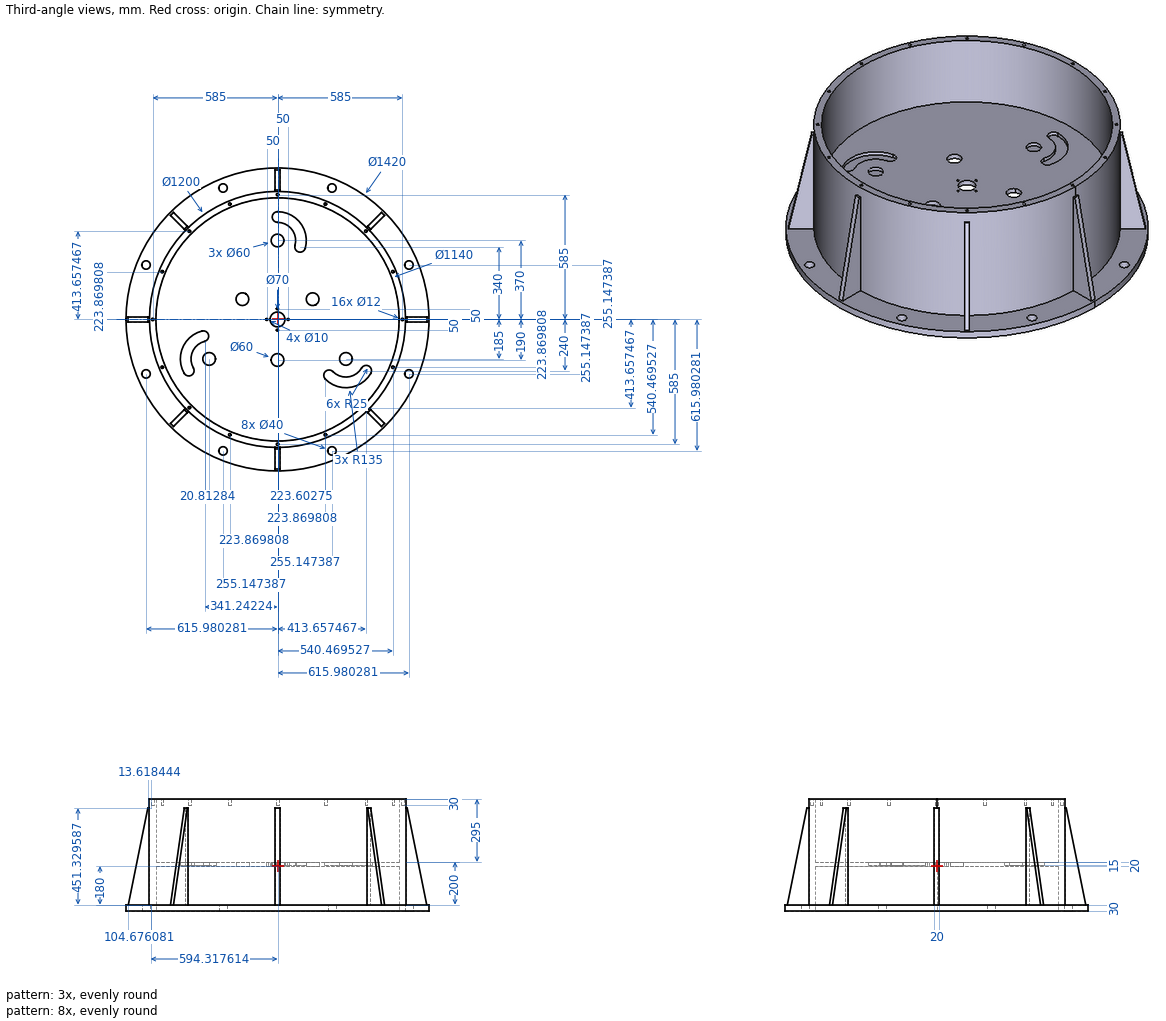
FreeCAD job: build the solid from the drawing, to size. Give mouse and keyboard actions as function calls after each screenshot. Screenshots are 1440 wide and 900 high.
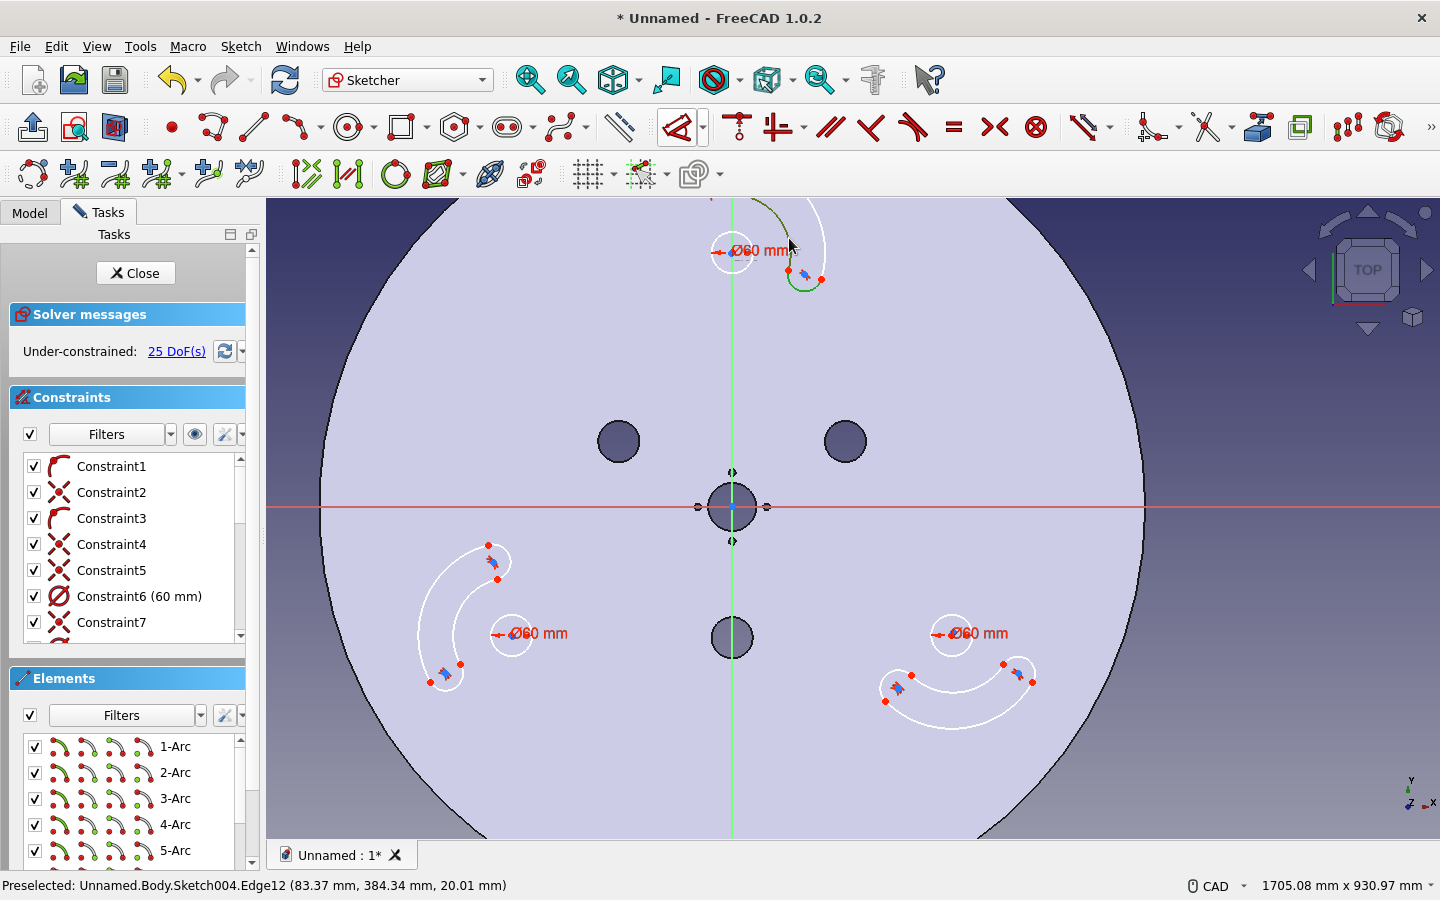
click(913, 128)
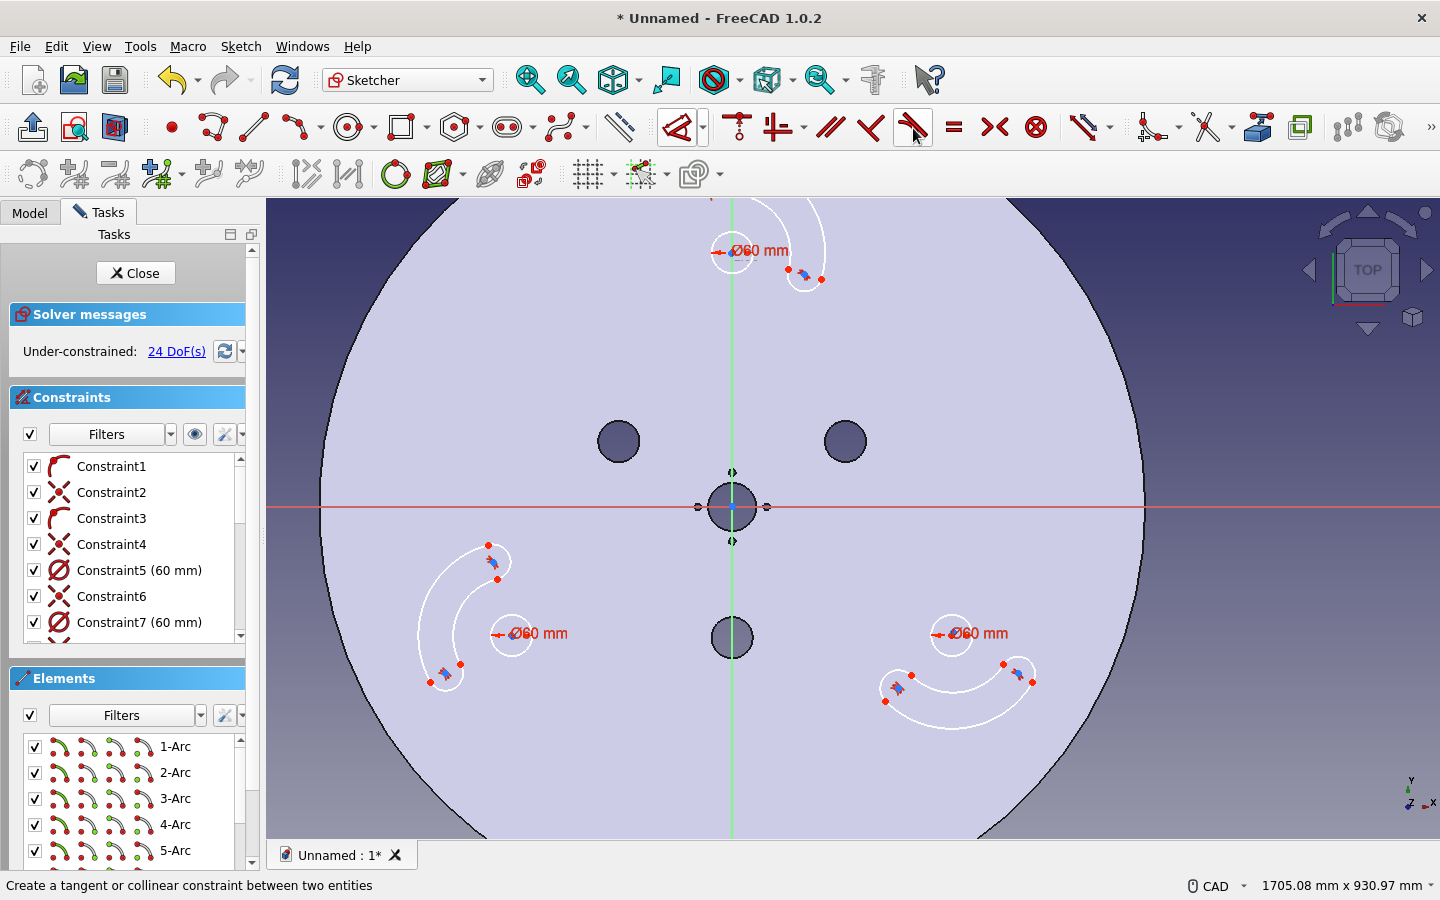
click(822, 228)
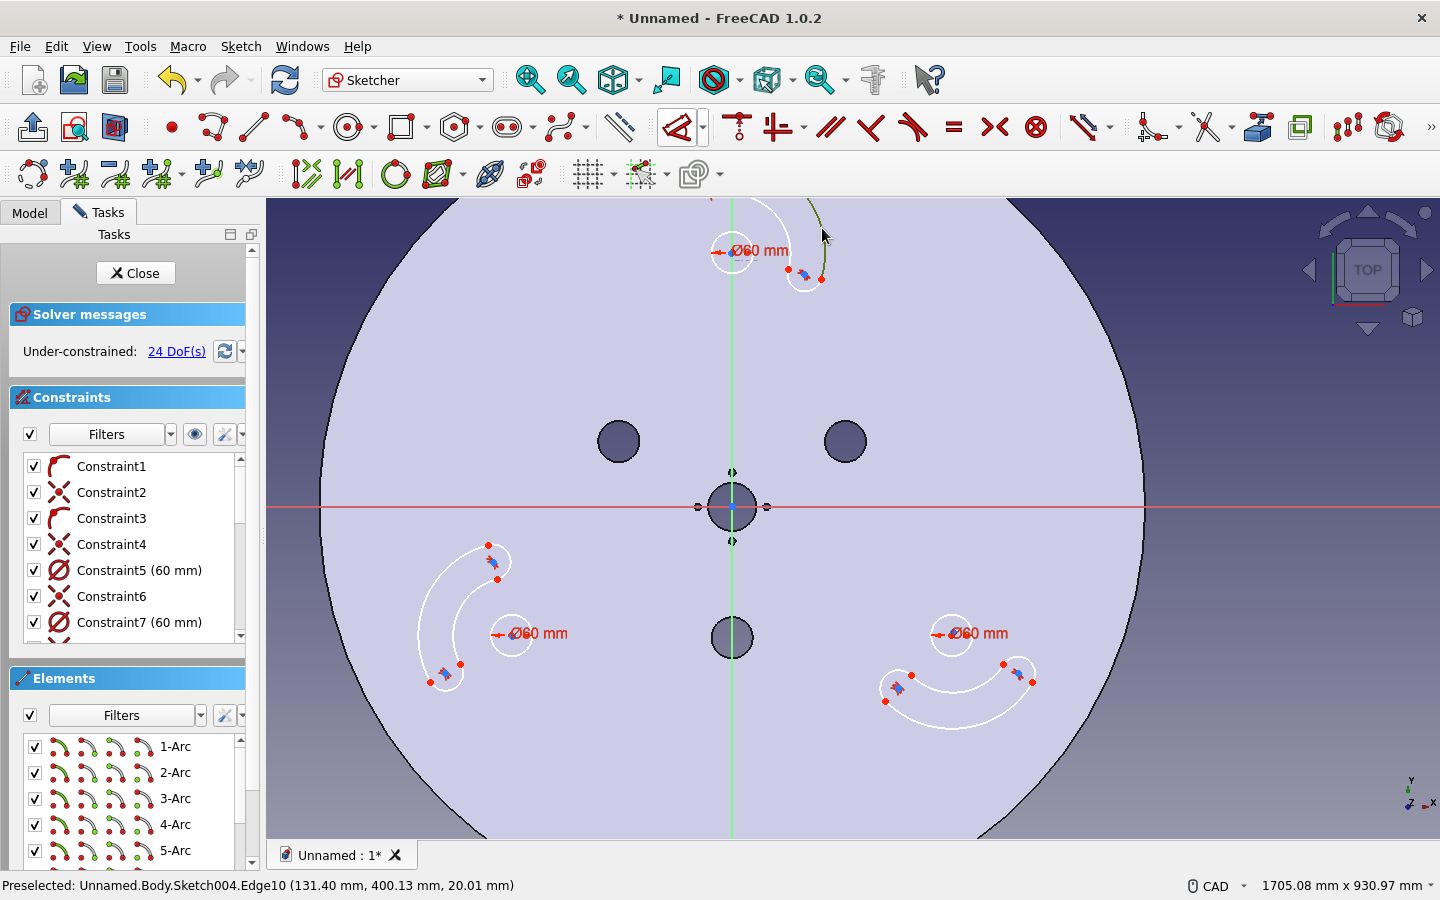
scroll(896, 672, down, 2)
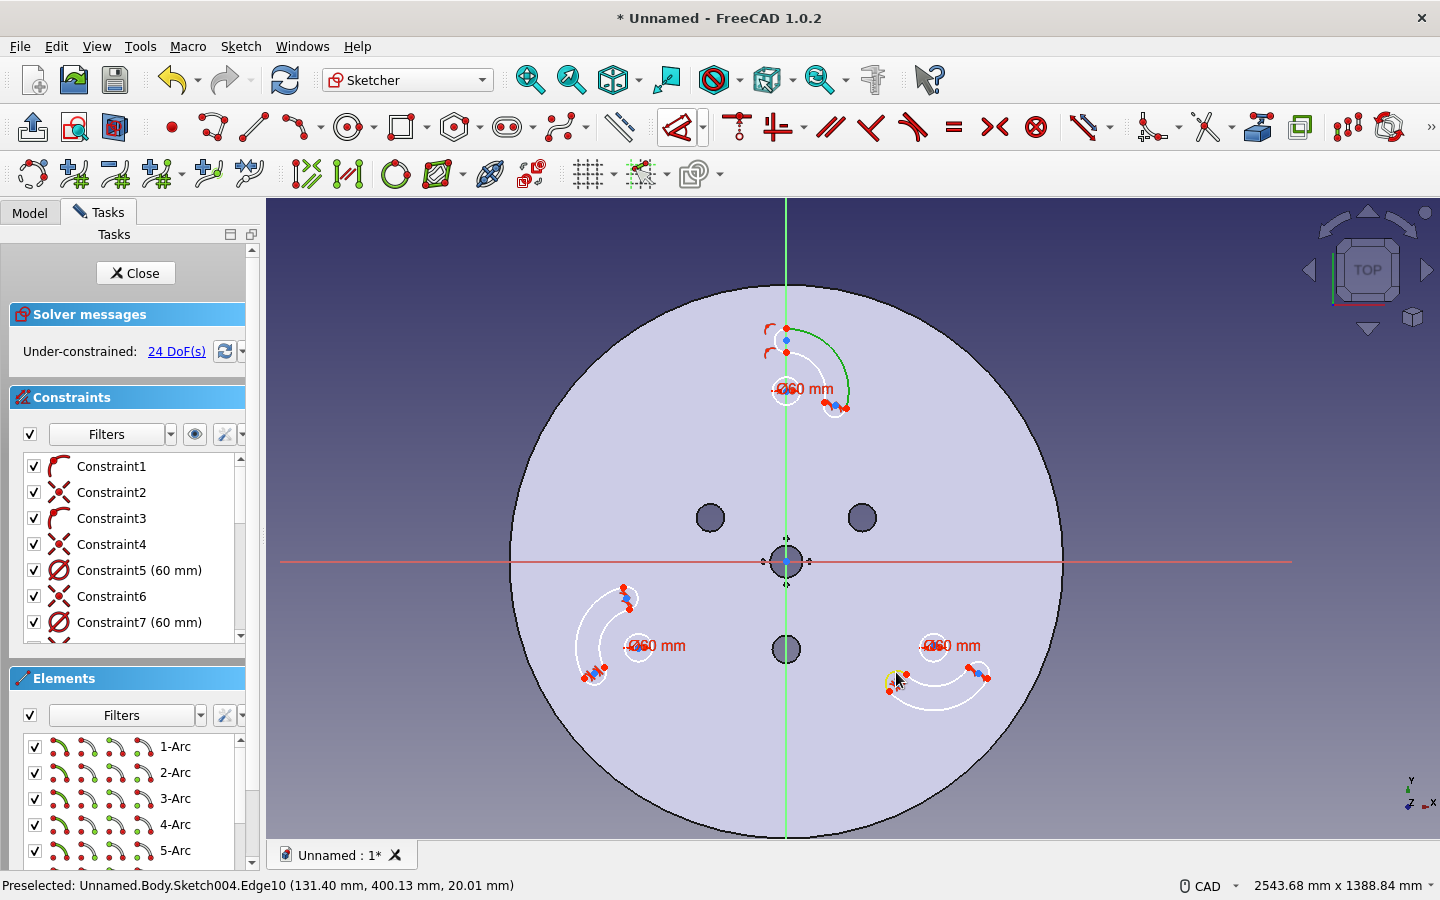
scroll(777, 334, up, 2)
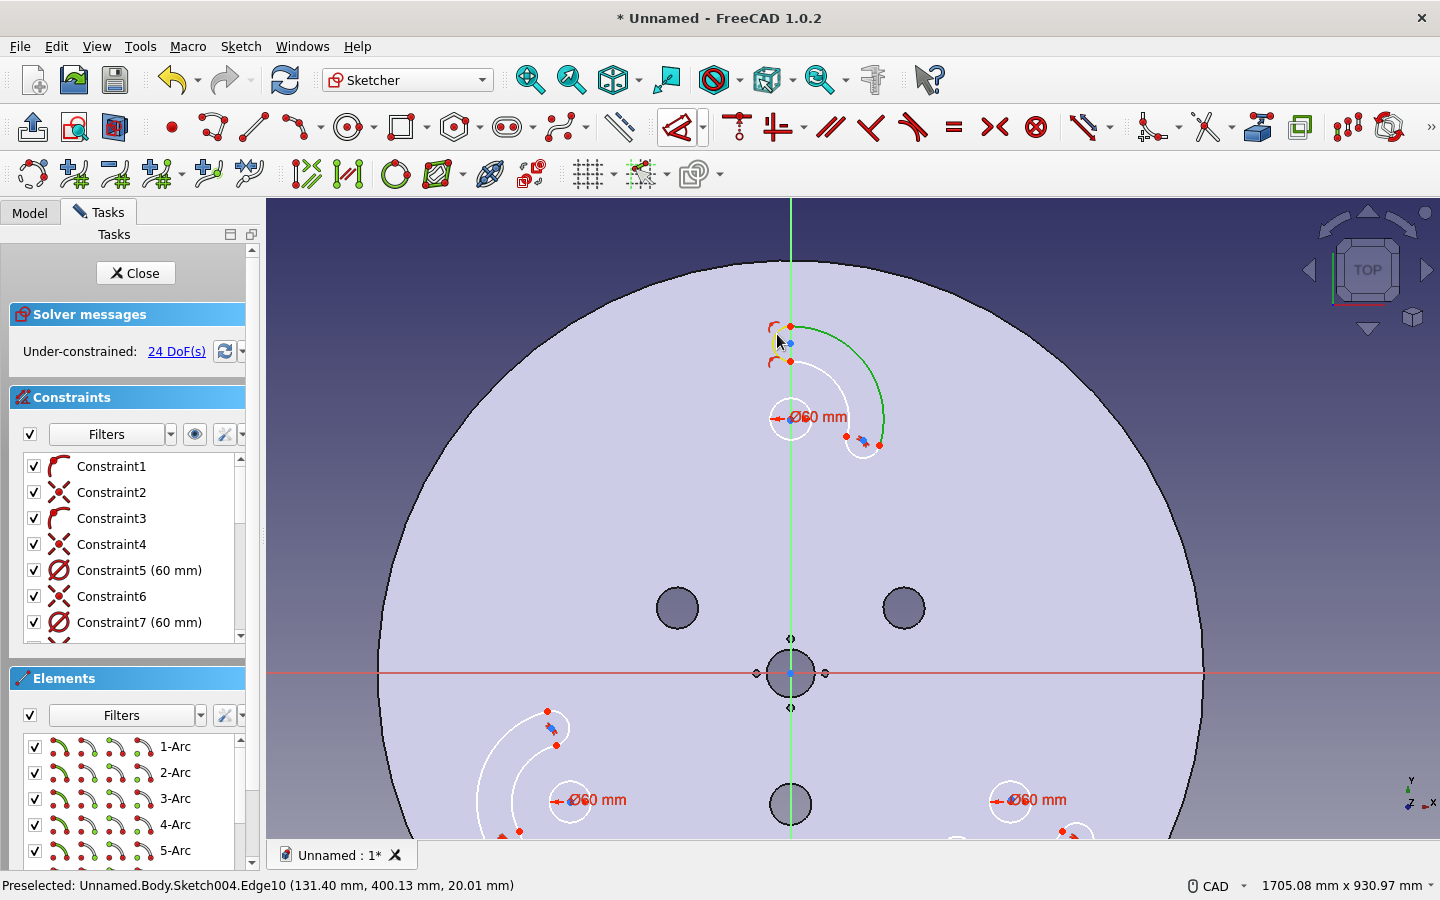
click(776, 334)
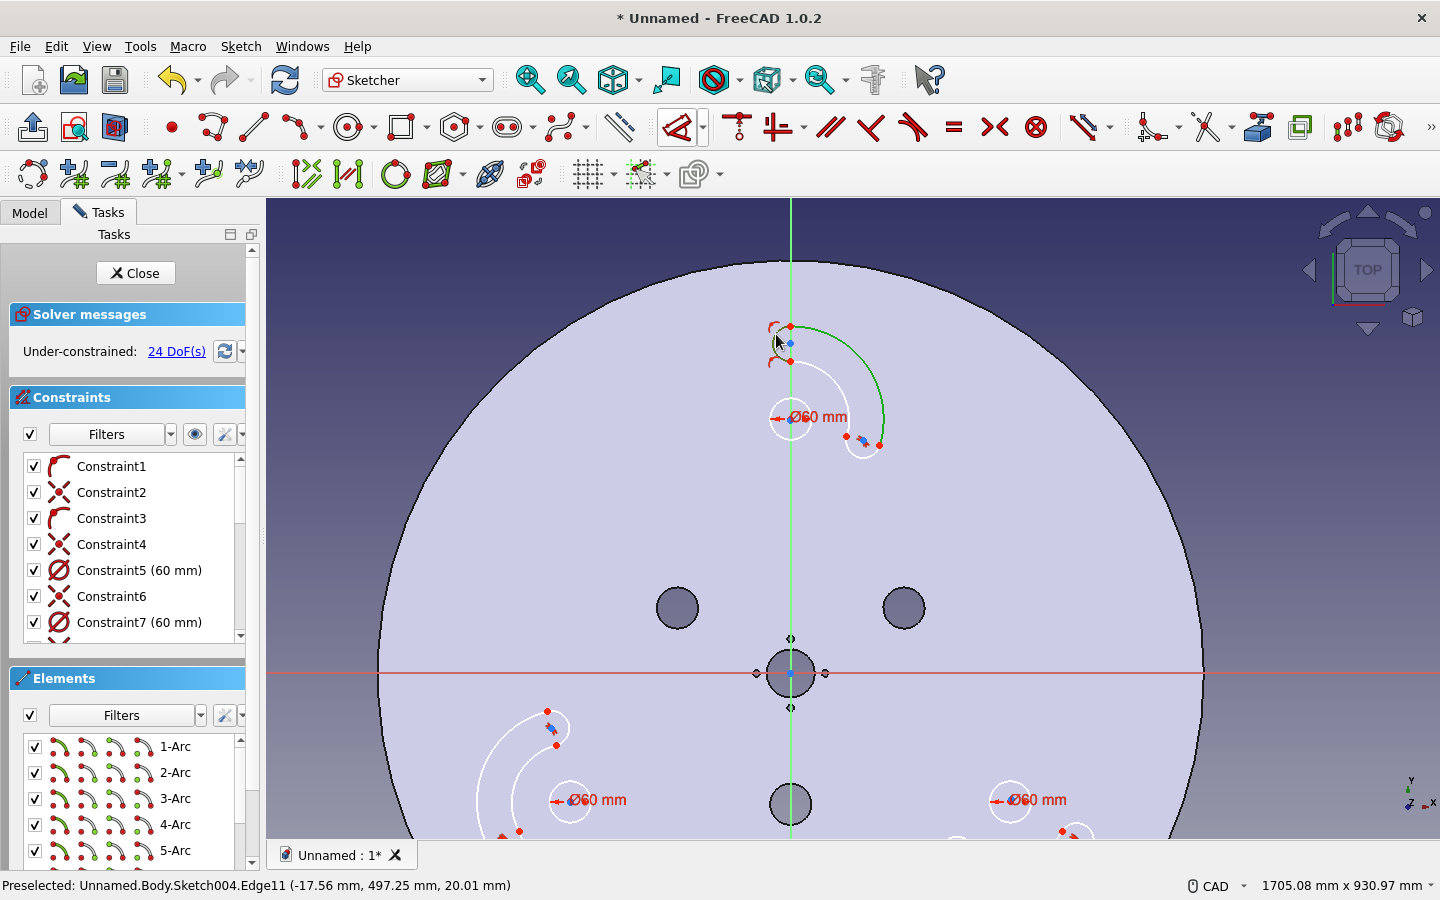
click(913, 128)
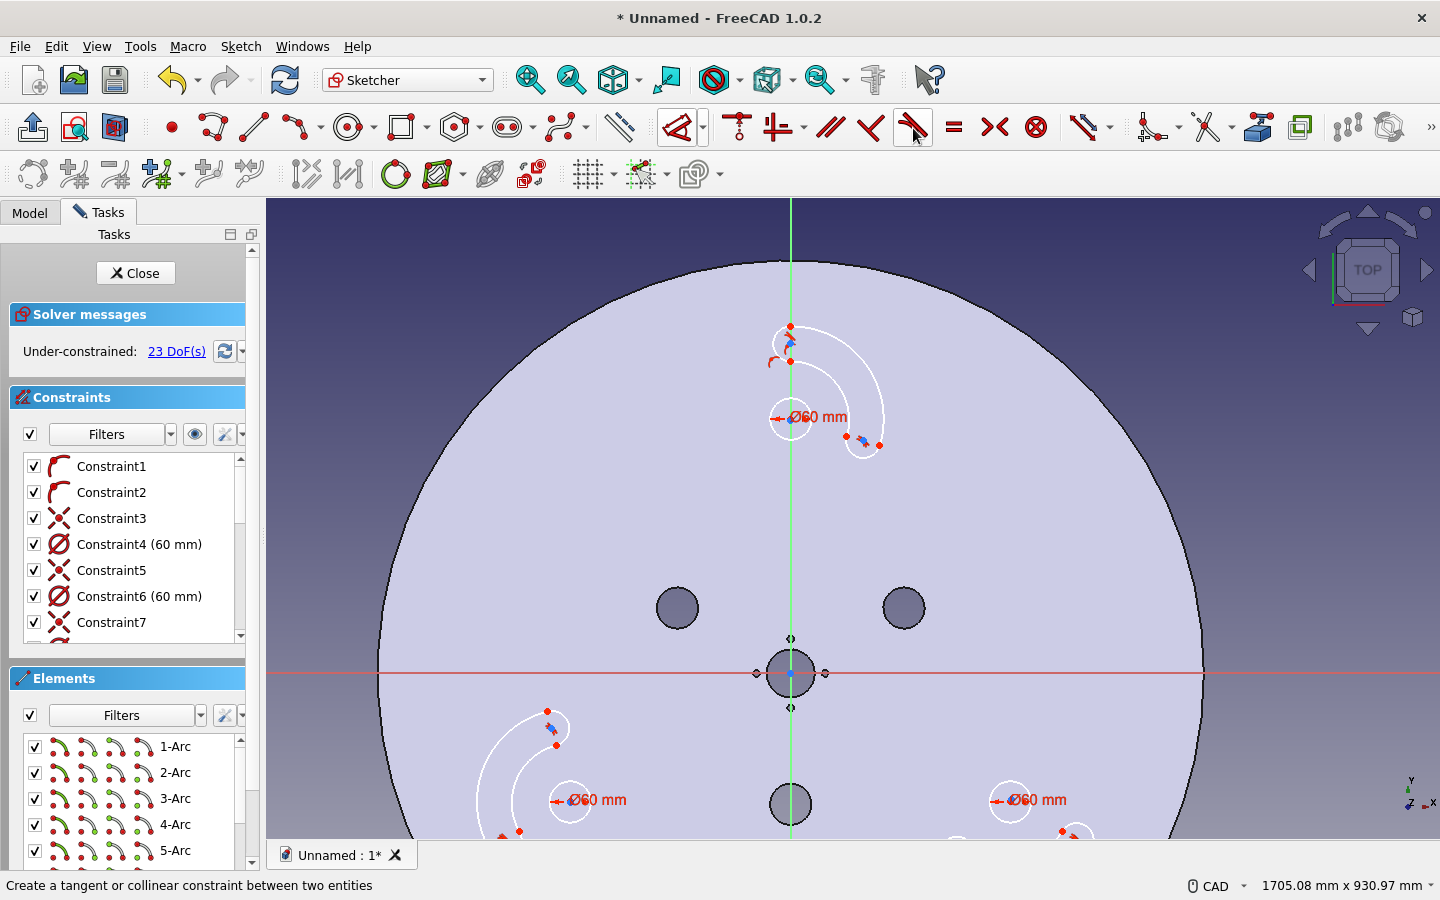
click(1025, 787)